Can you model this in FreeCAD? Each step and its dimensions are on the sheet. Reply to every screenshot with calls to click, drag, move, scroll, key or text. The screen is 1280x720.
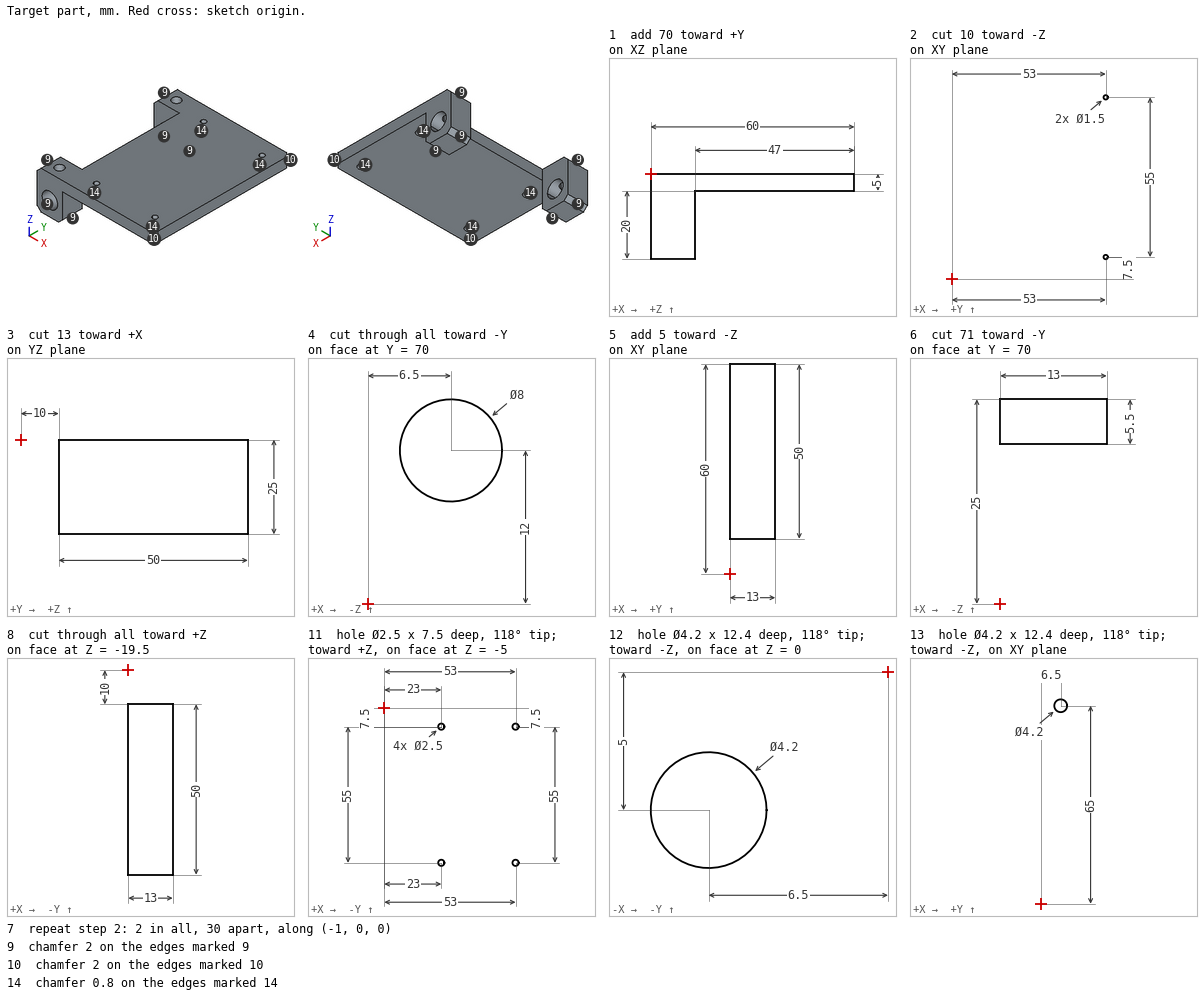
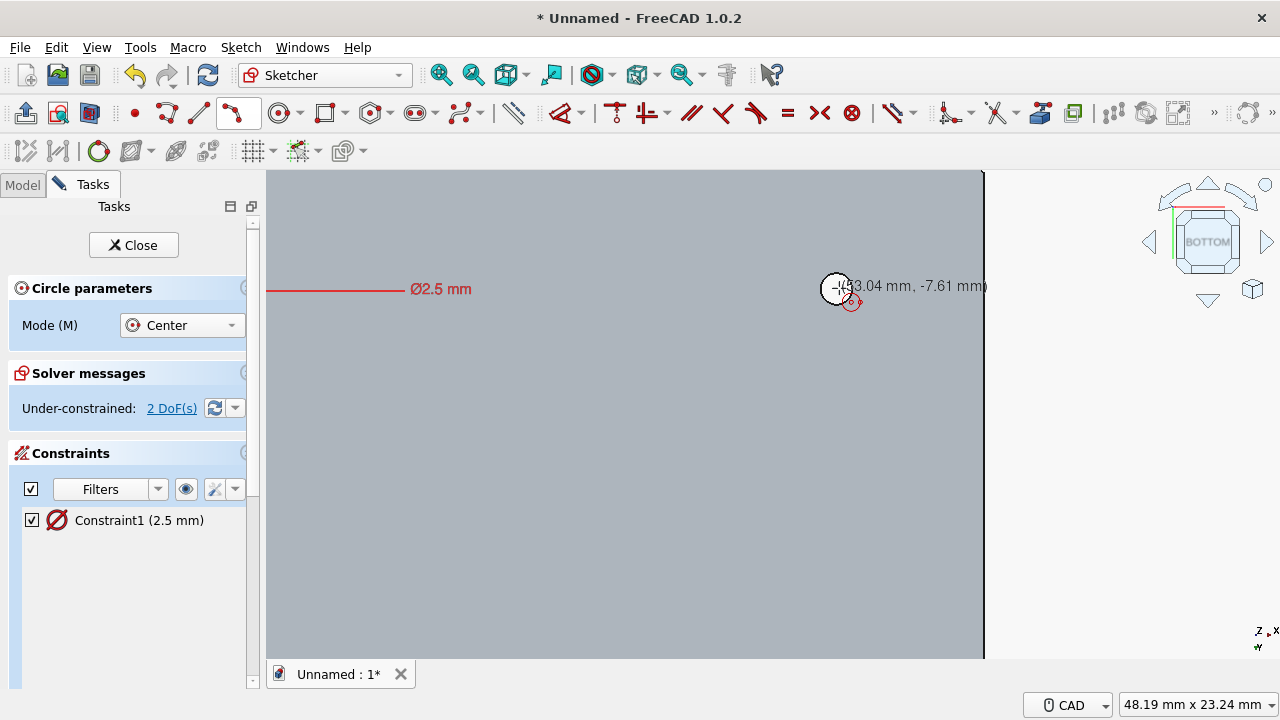
scroll(840, 288, down, 7)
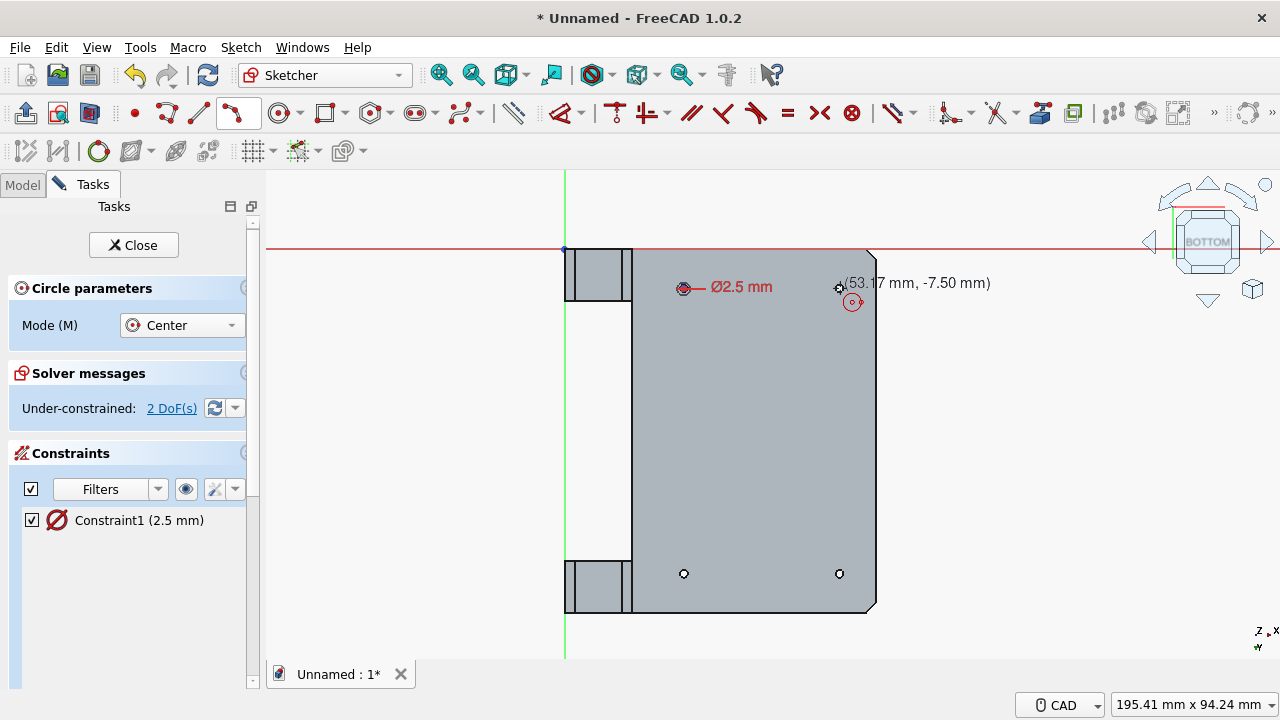
click(840, 288)
move(844, 284)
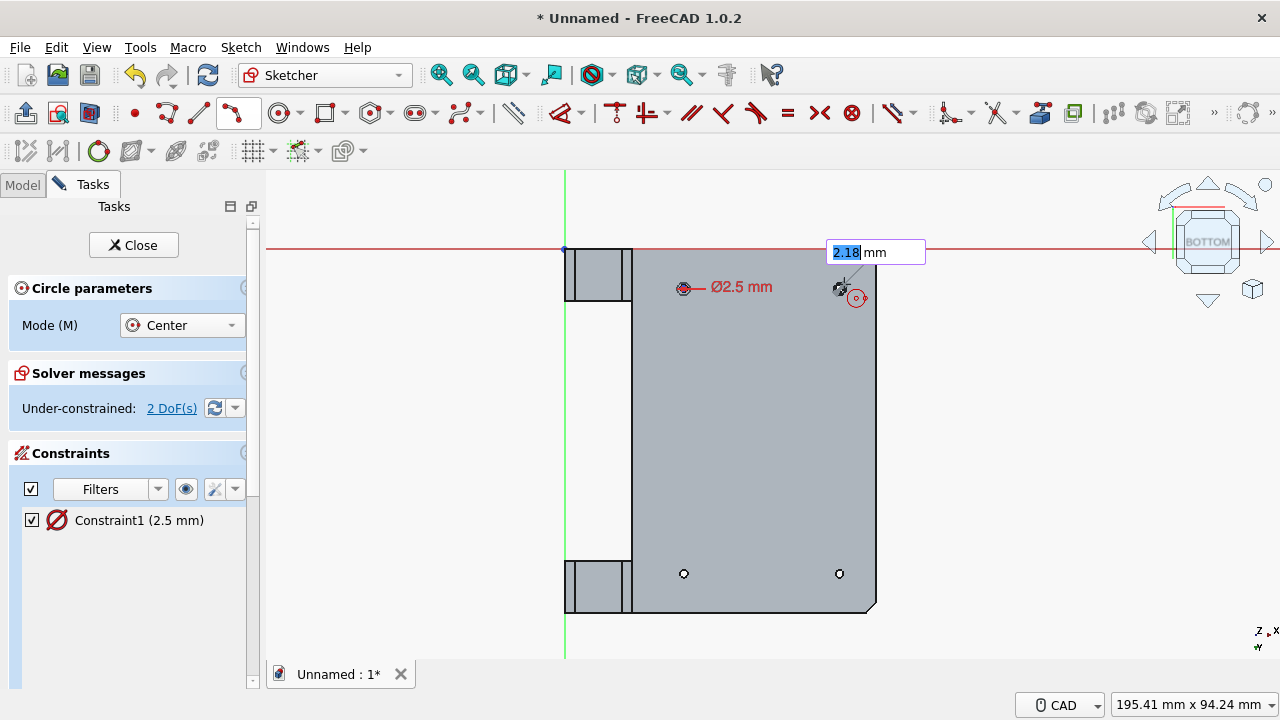
text(2.5)
key(Return)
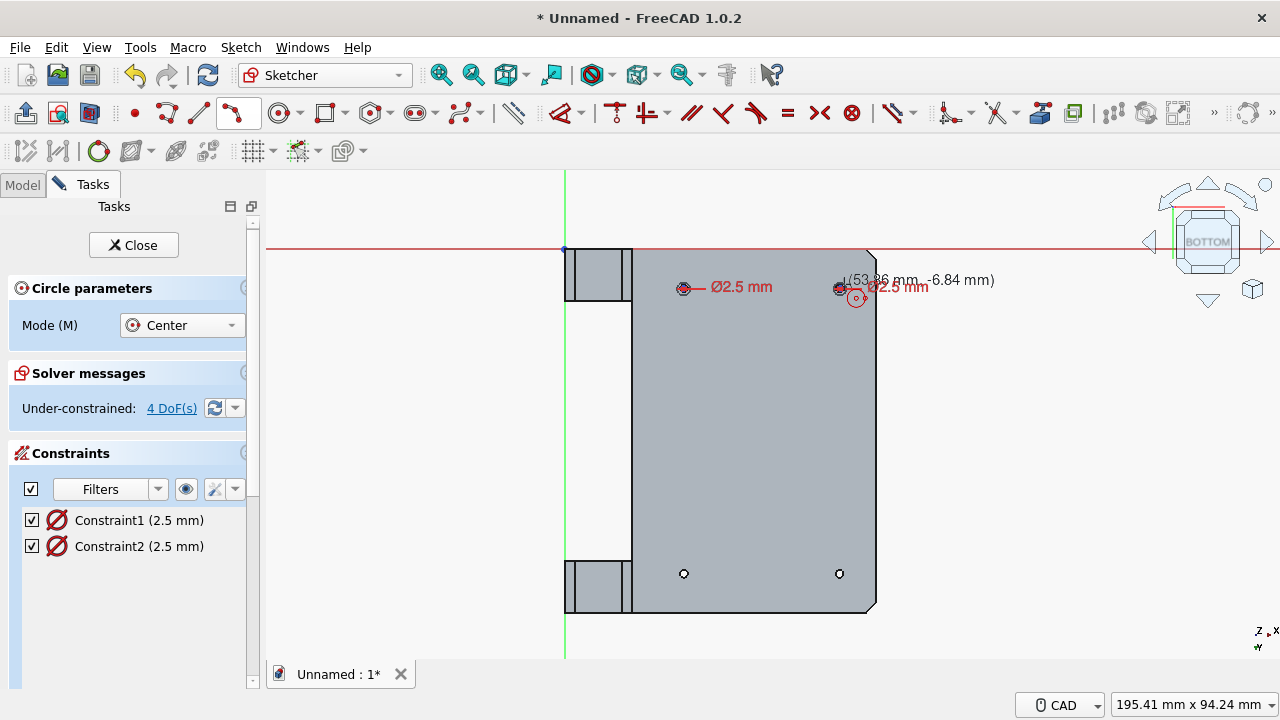
scroll(840, 574, up, 7)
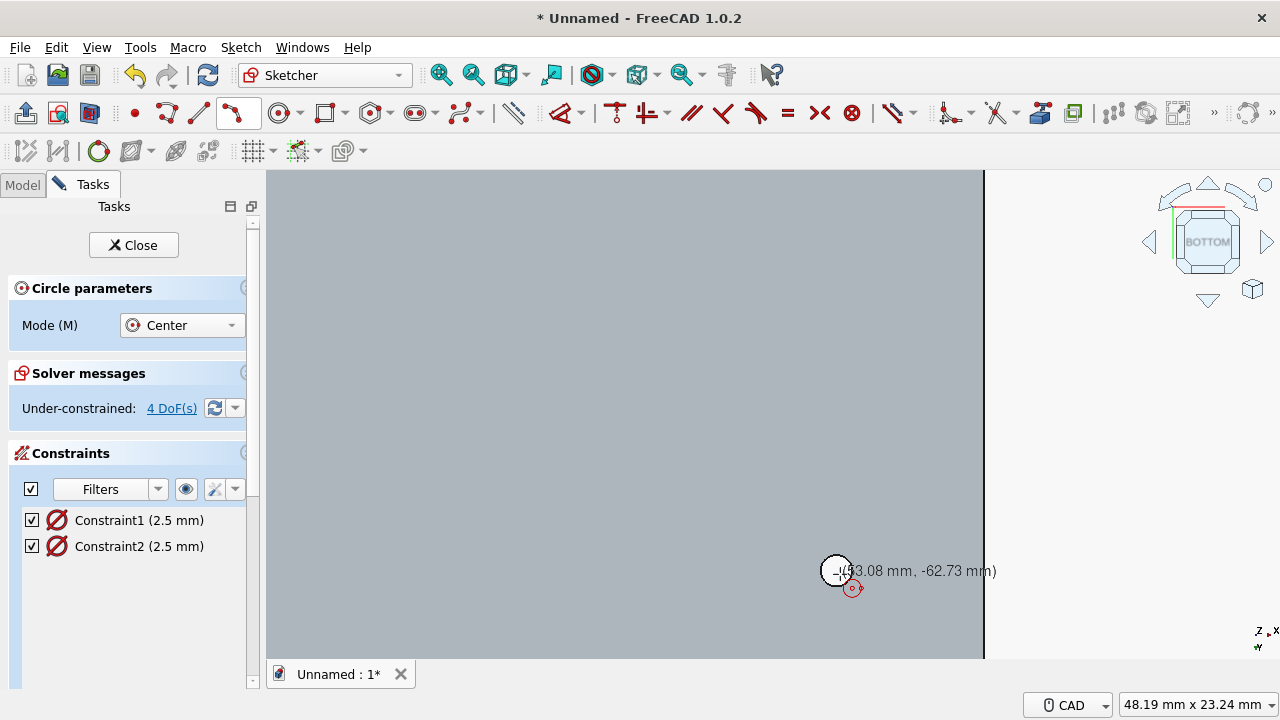
scroll(840, 574, down, 7)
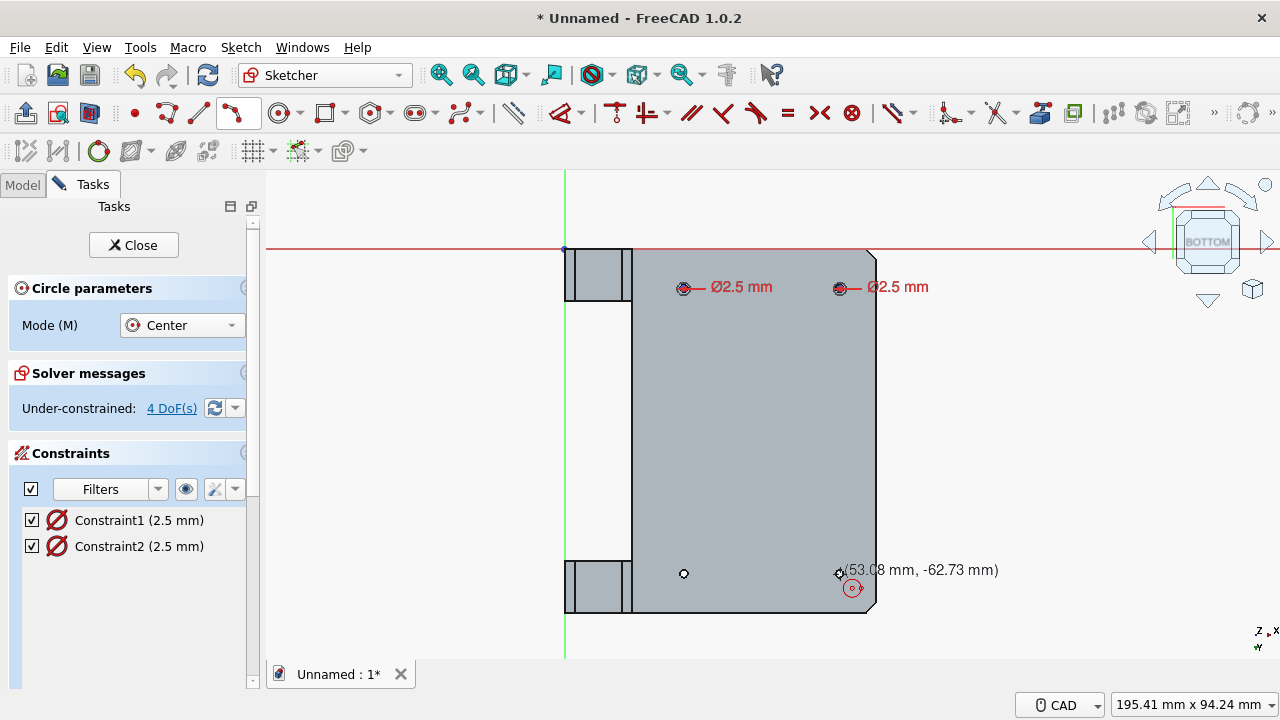
click(840, 574)
move(844, 569)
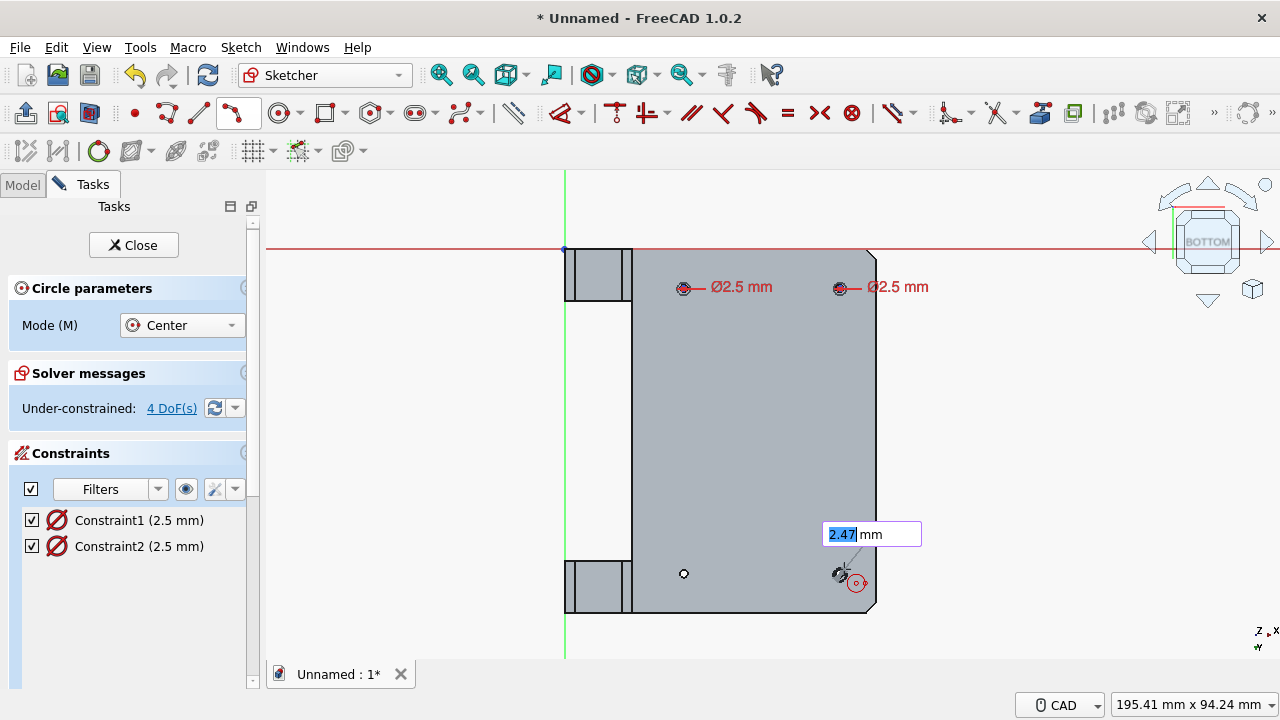
text(2.5)
key(Return)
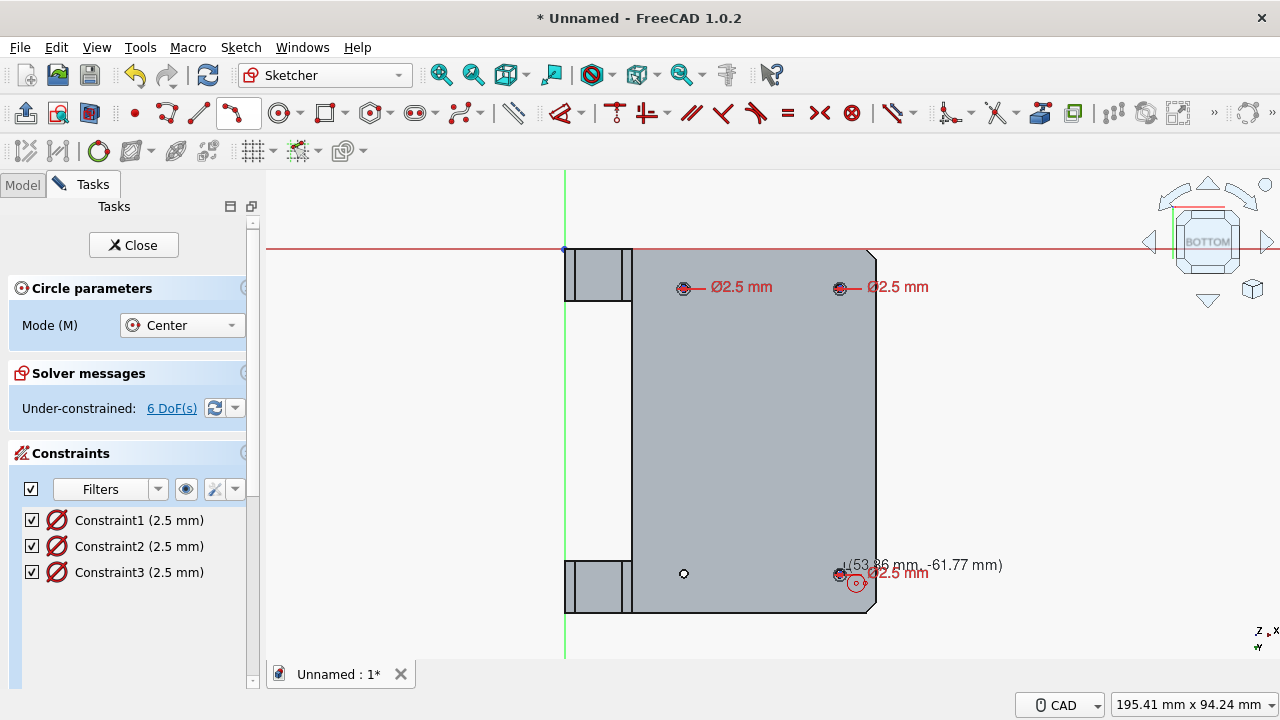
scroll(684, 574, up, 7)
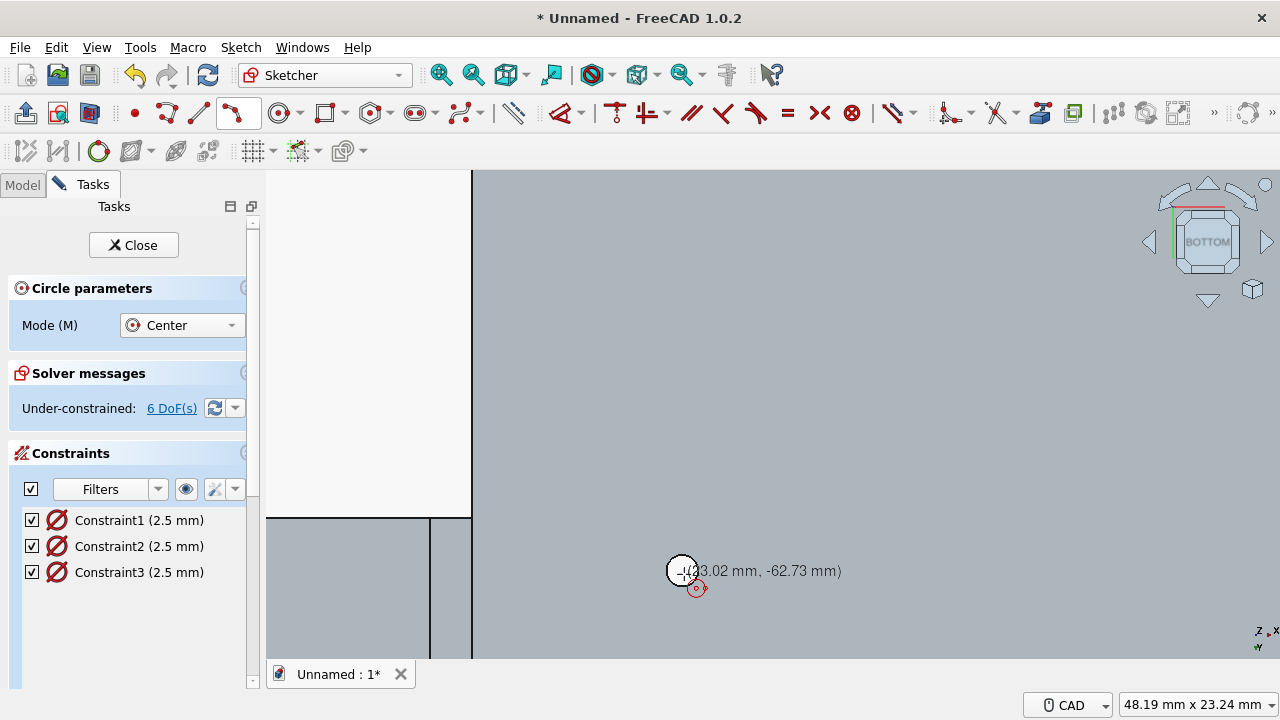
scroll(683, 574, down, 7)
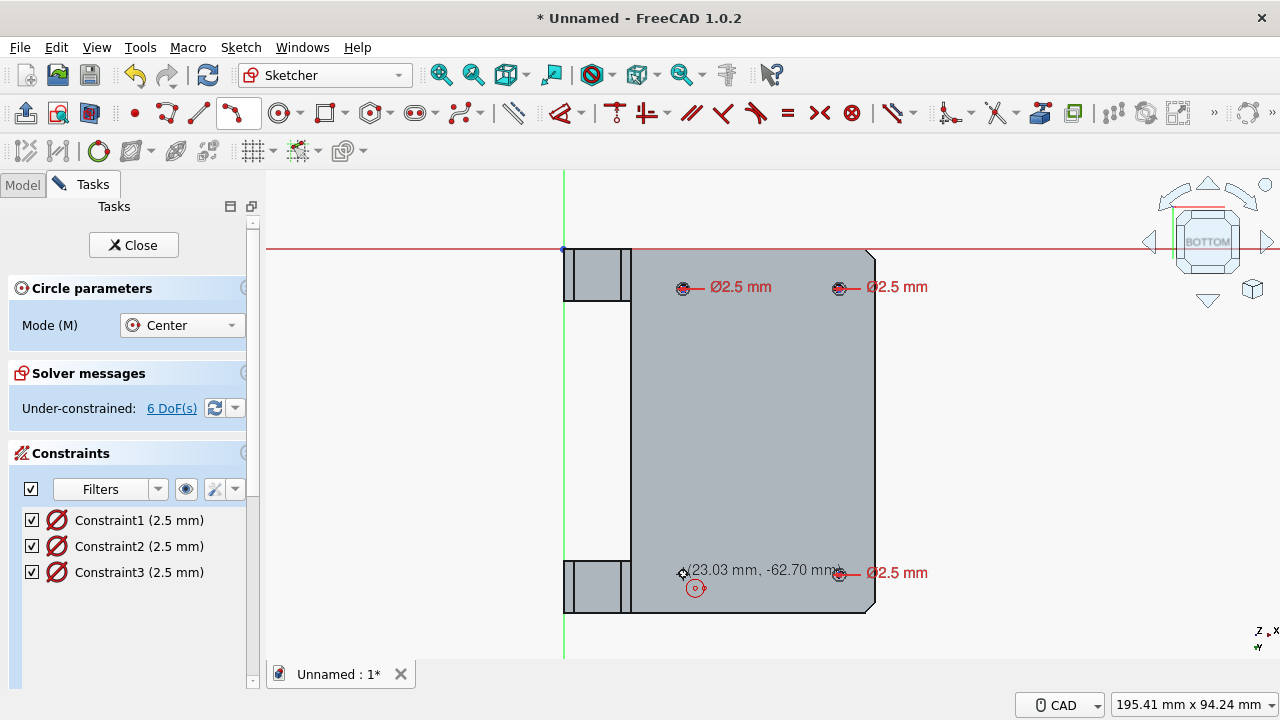
click(683, 574)
move(688, 569)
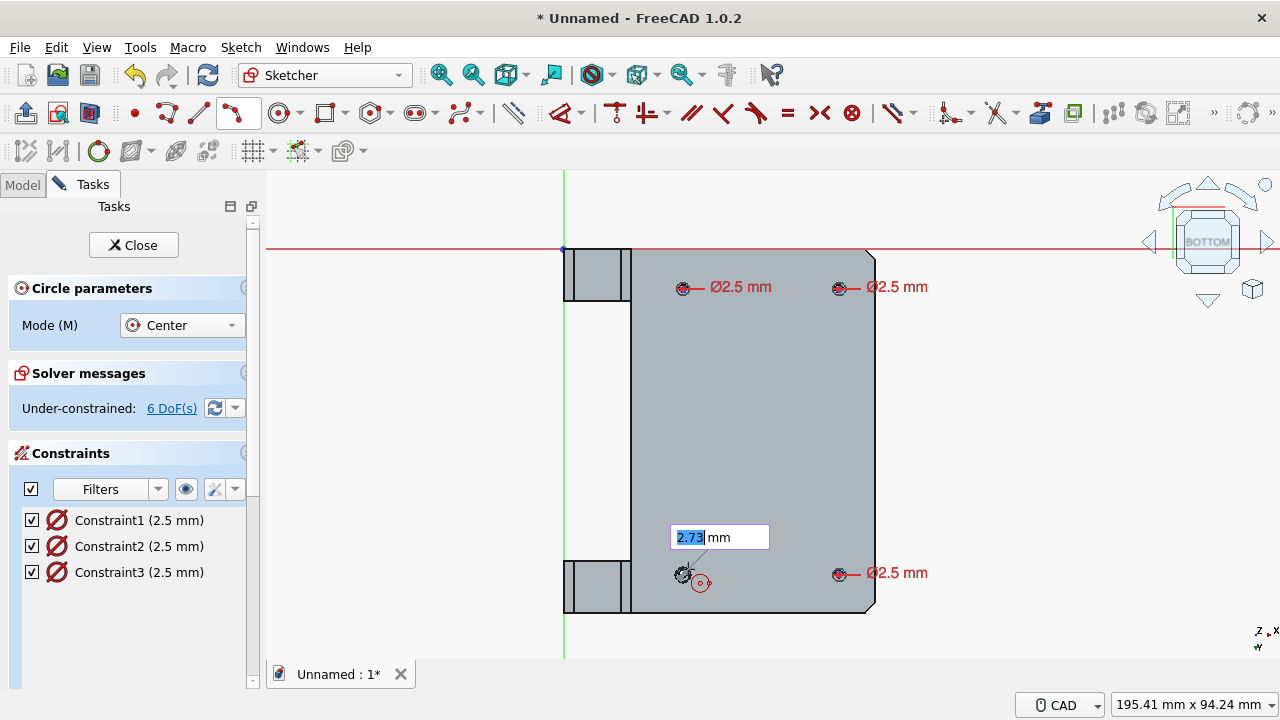
text(2.5)
key(Return)
key(Escape)